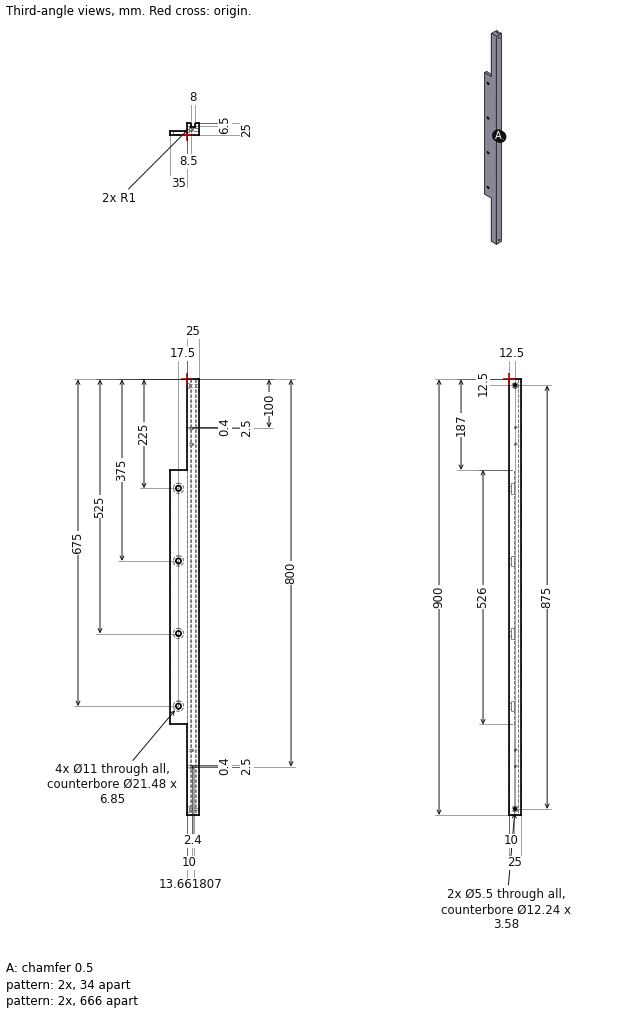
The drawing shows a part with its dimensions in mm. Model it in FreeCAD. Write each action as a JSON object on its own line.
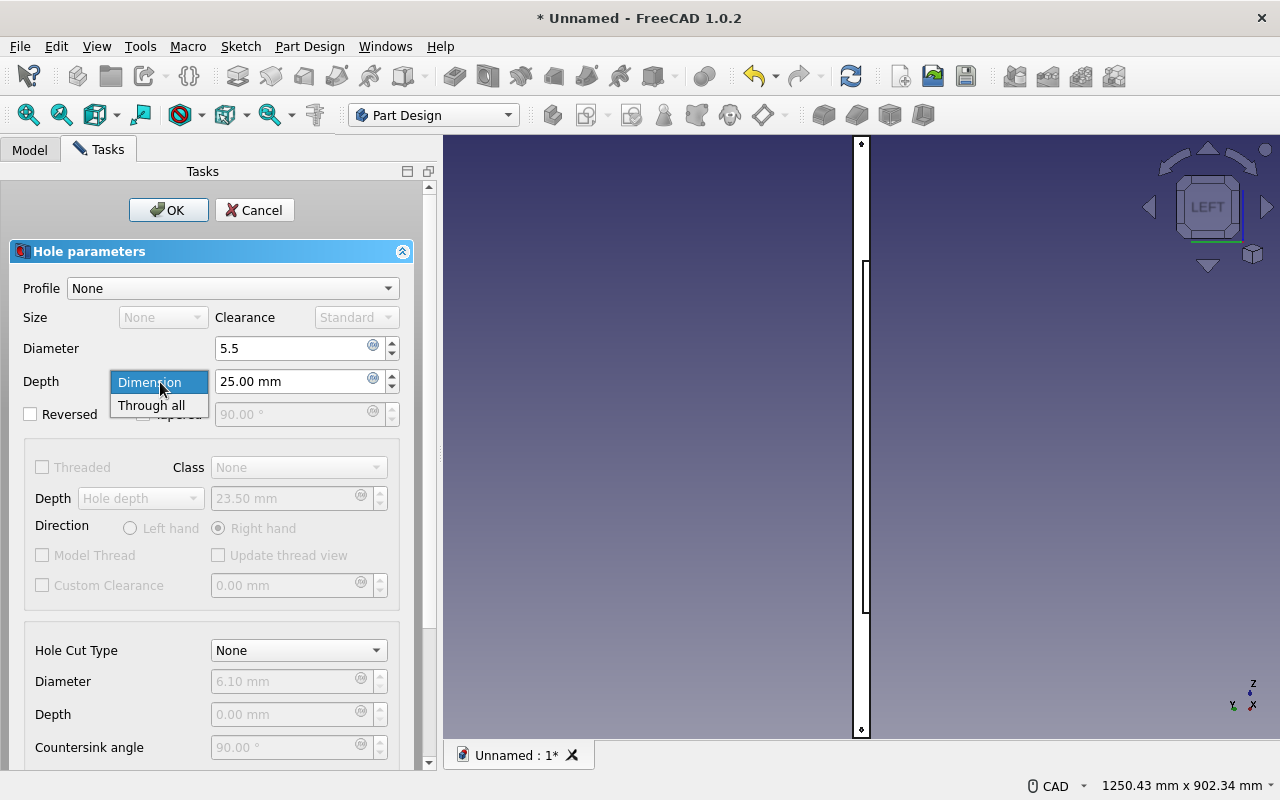
{"action": "left_click", "coordinate": [158, 406]}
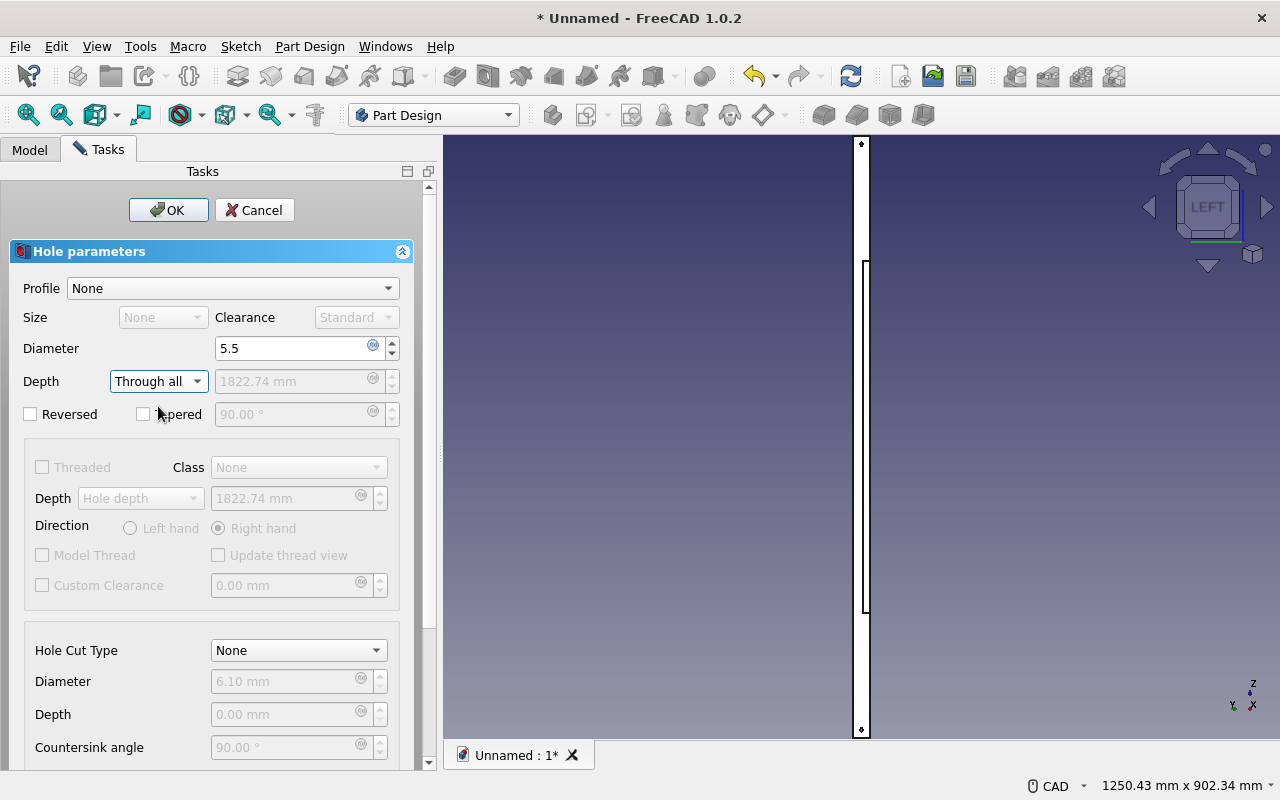
{"action": "left_click", "coordinate": [300, 650]}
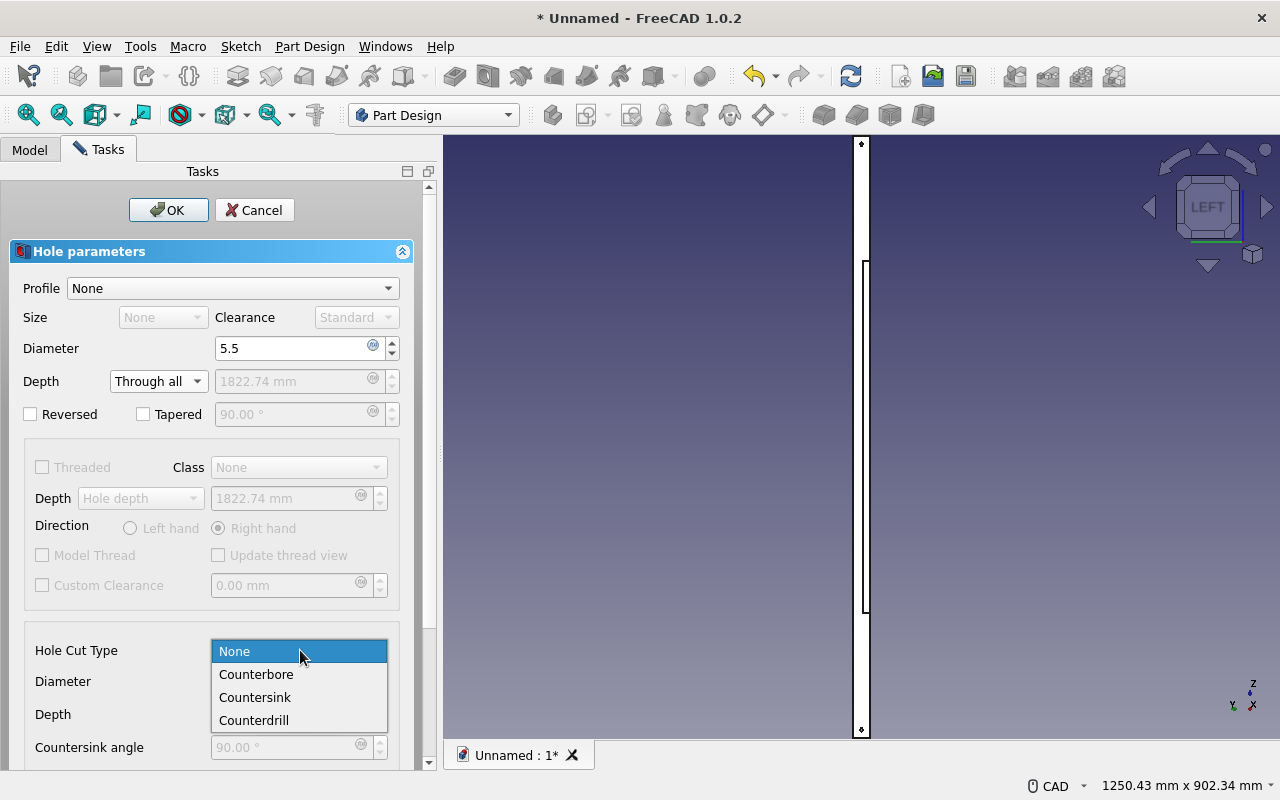
{"action": "left_click", "coordinate": [298, 674]}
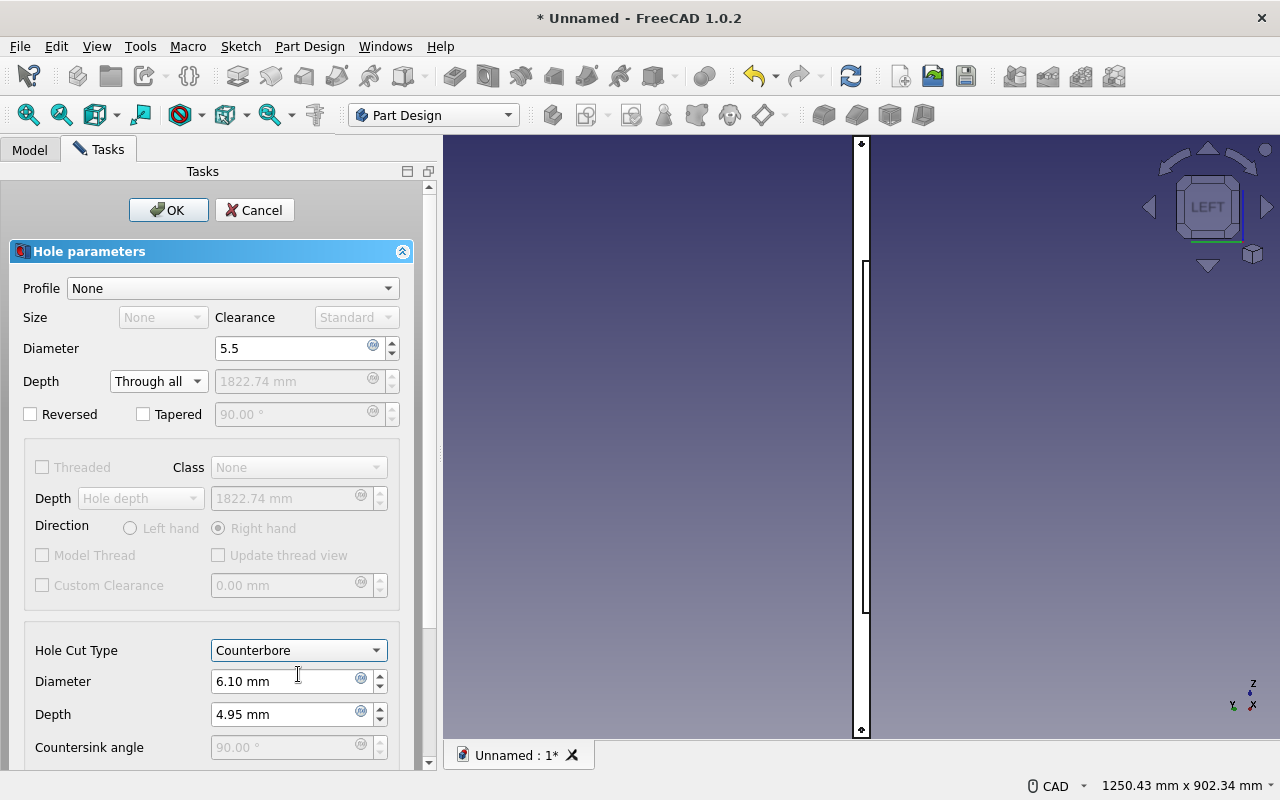
{"action": "triple_click", "coordinate": [292, 682]}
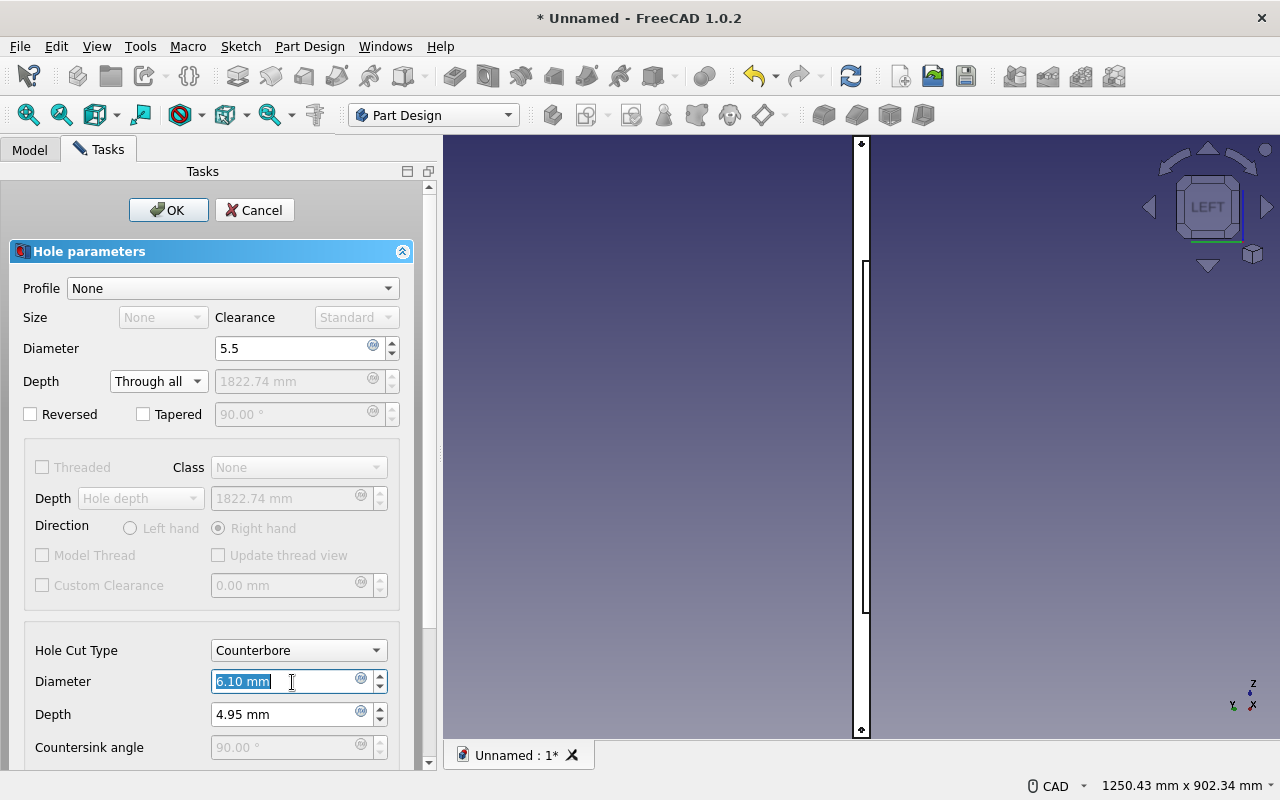
{"action": "type", "text": "12.24"}
{"action": "key", "text": "Tab"}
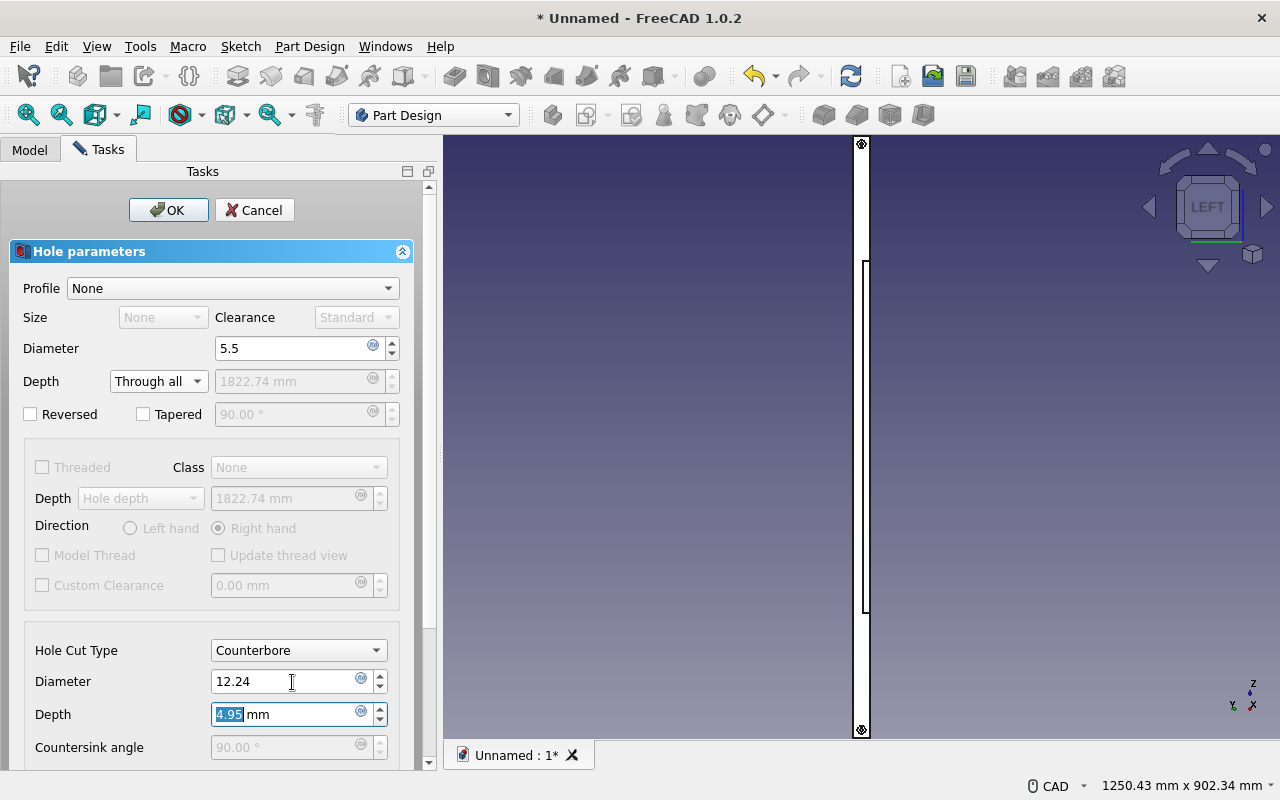
{"action": "type", "text": "3.58"}
{"action": "key", "text": "Tab"}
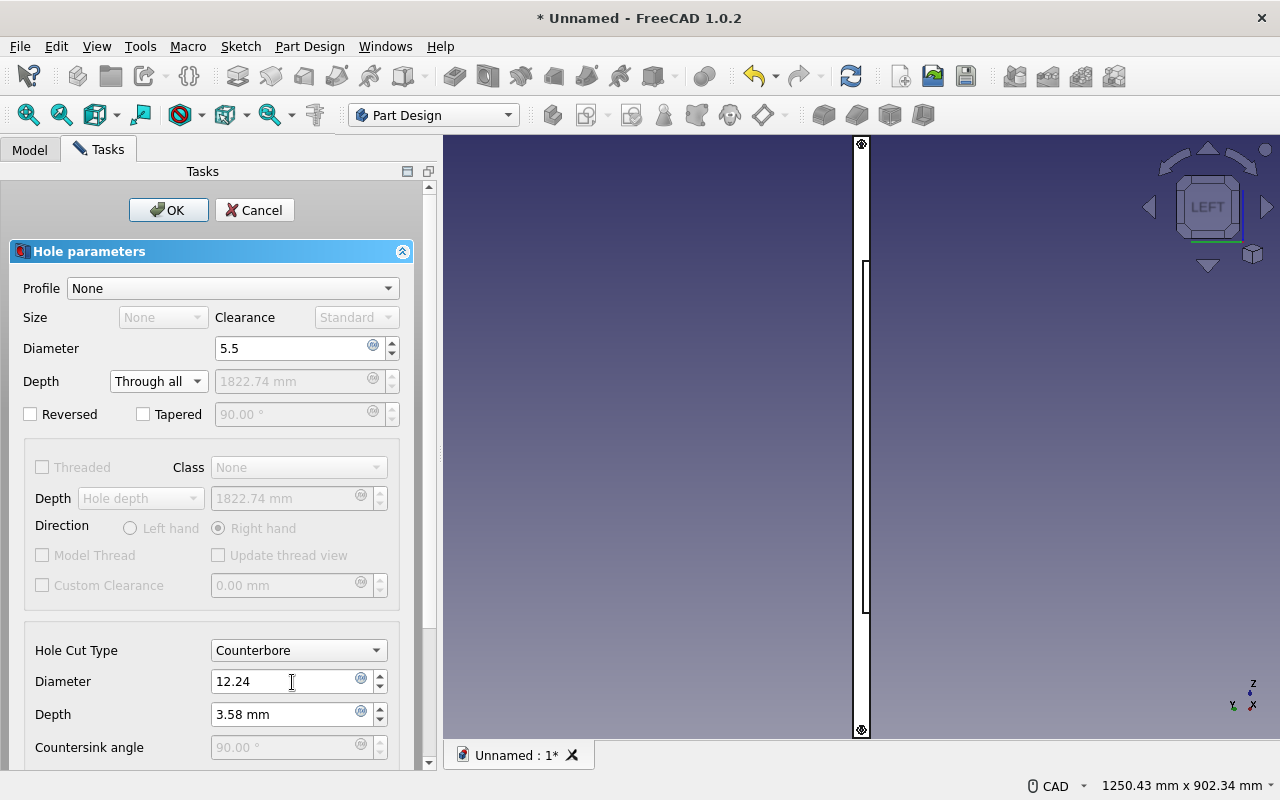
{"action": "left_click", "coordinate": [169, 210]}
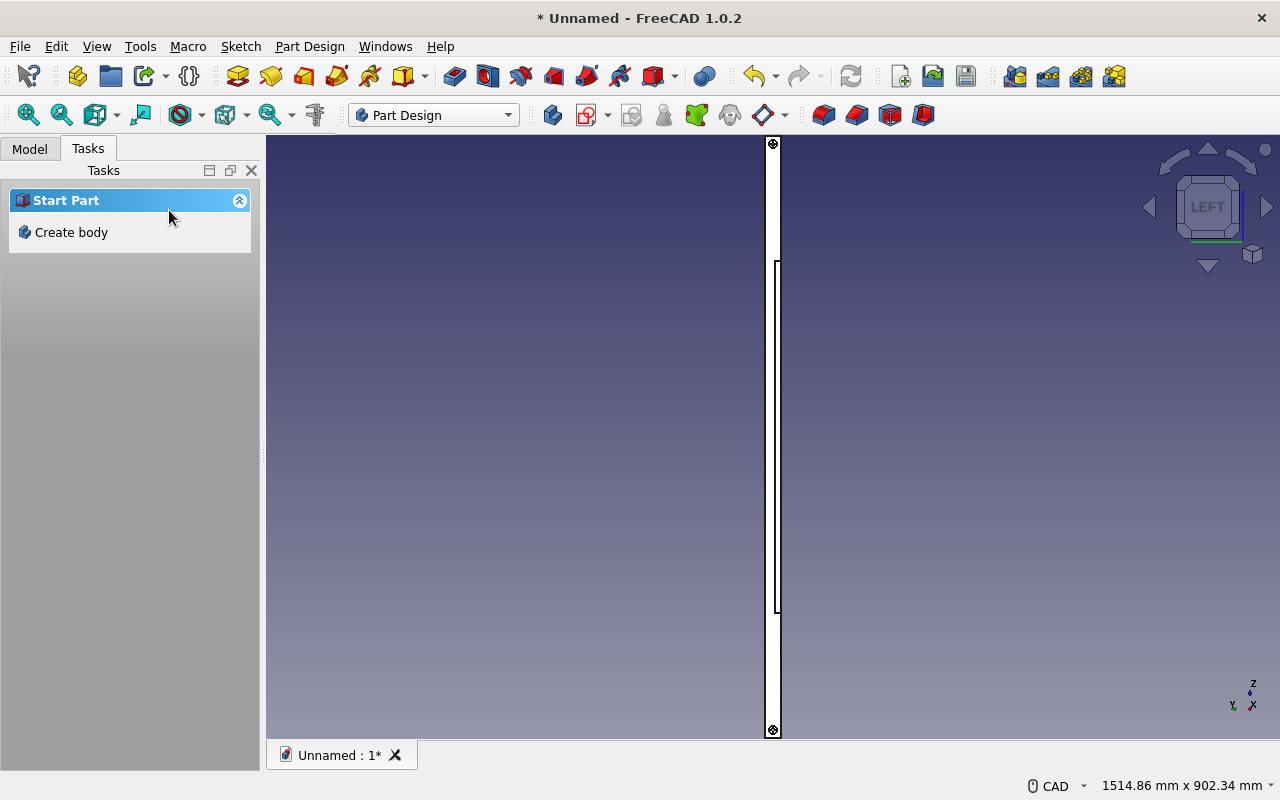
{"action": "left_click", "coordinate": [30, 148]}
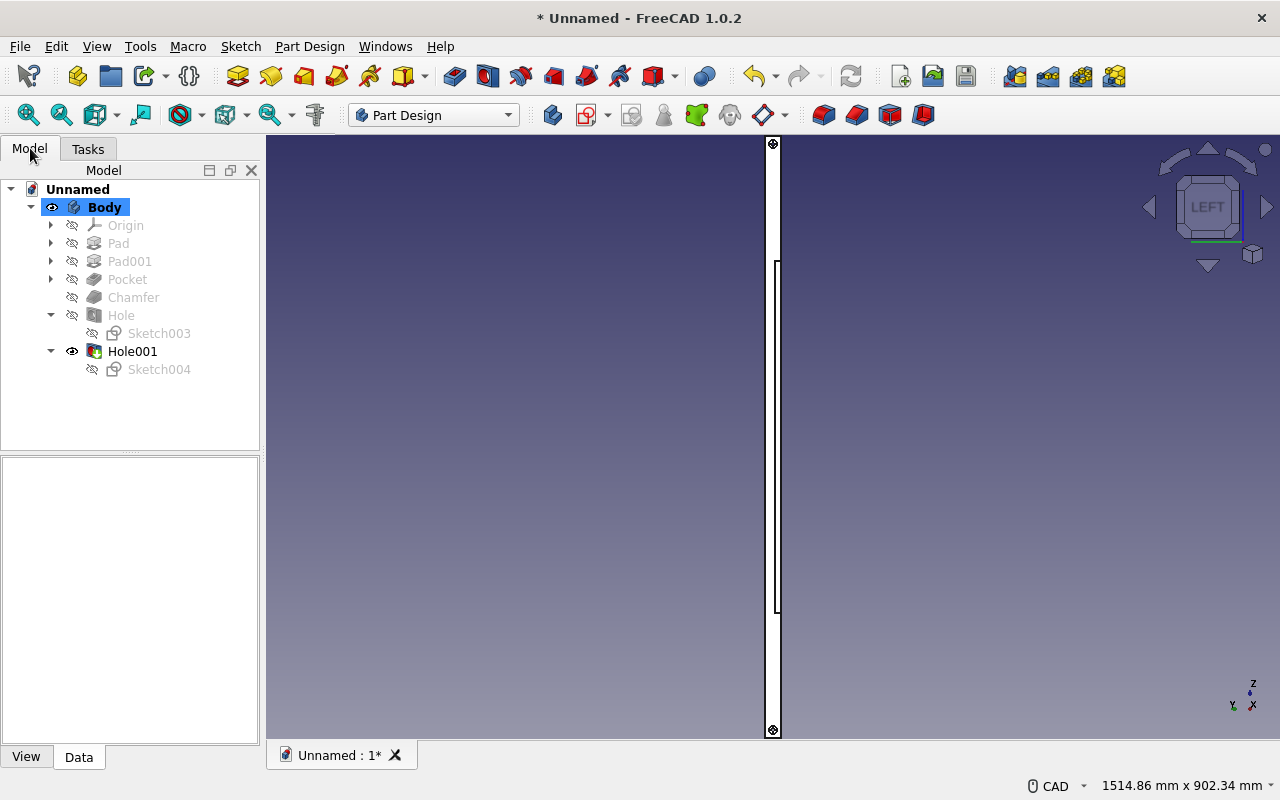
{"action": "left_click", "coordinate": [51, 225]}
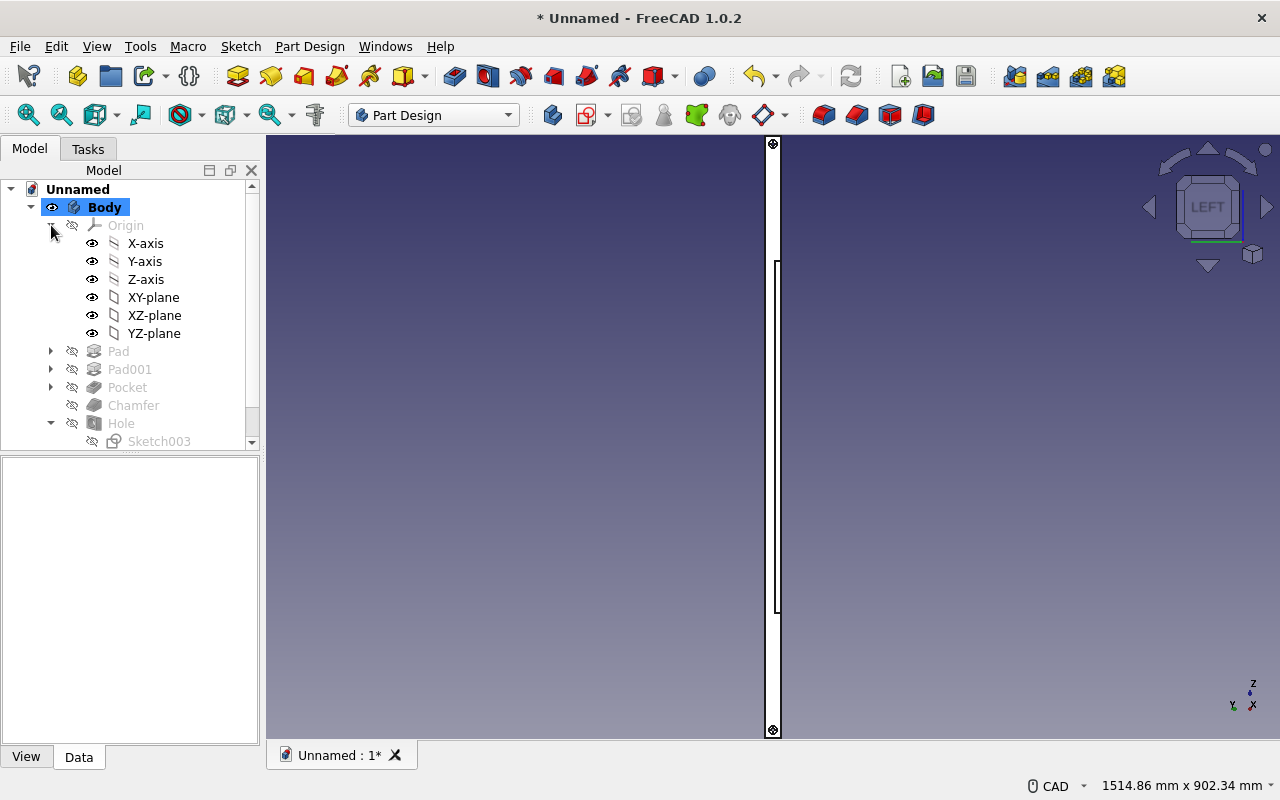
{"action": "left_click", "coordinate": [137, 315]}